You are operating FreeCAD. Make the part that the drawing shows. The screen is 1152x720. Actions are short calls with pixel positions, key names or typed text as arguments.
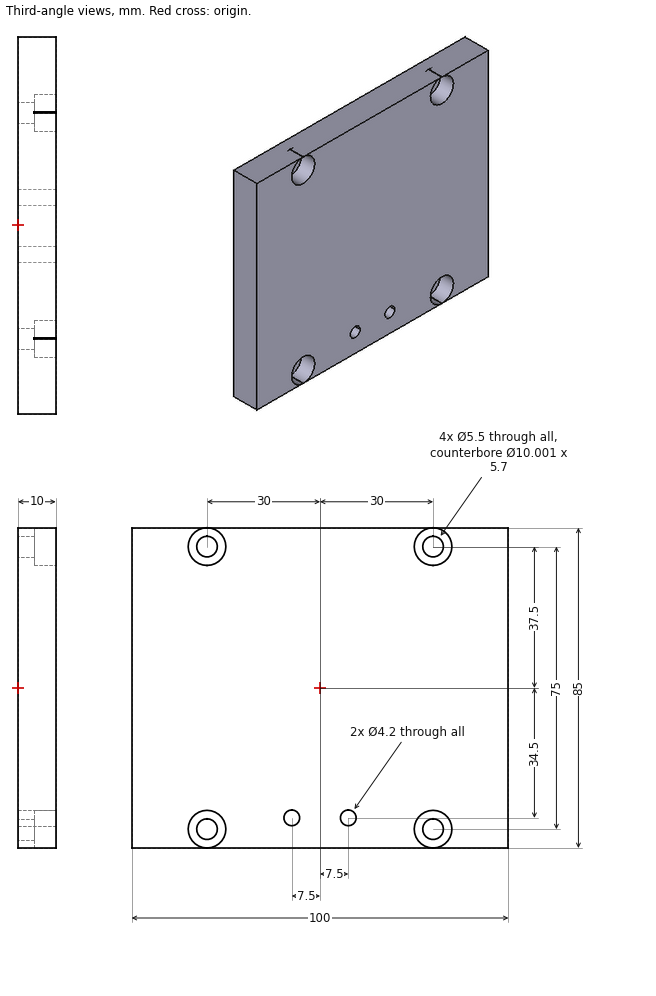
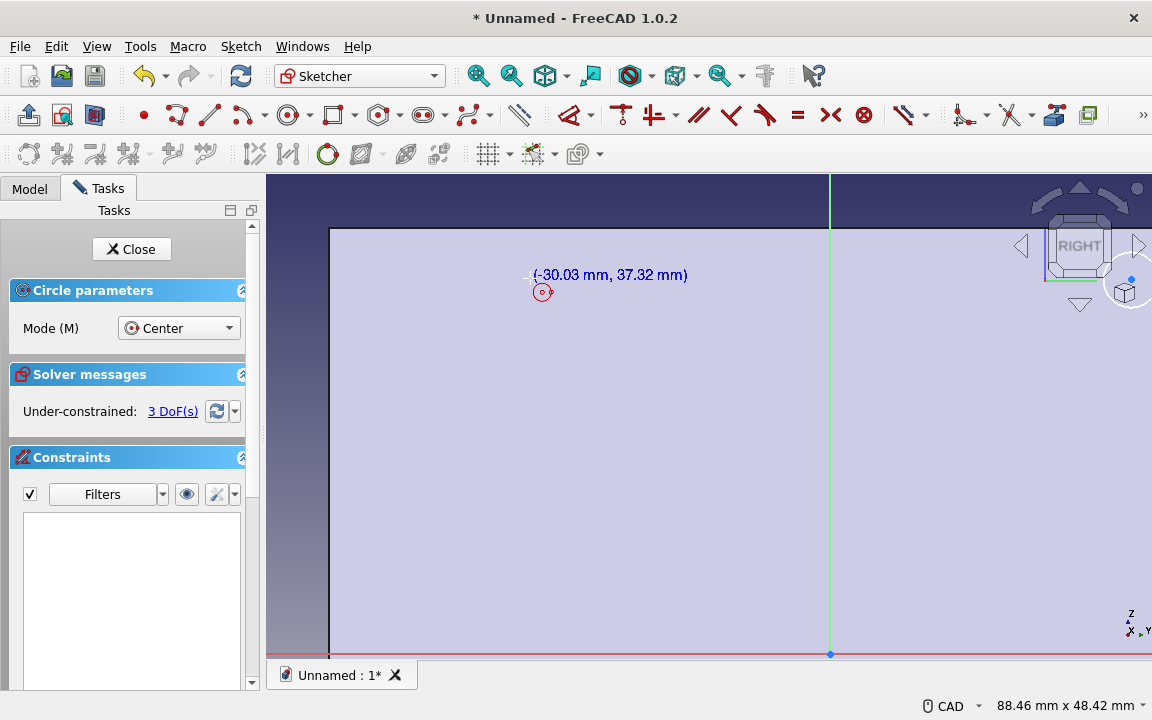
click(530, 279)
click(549, 259)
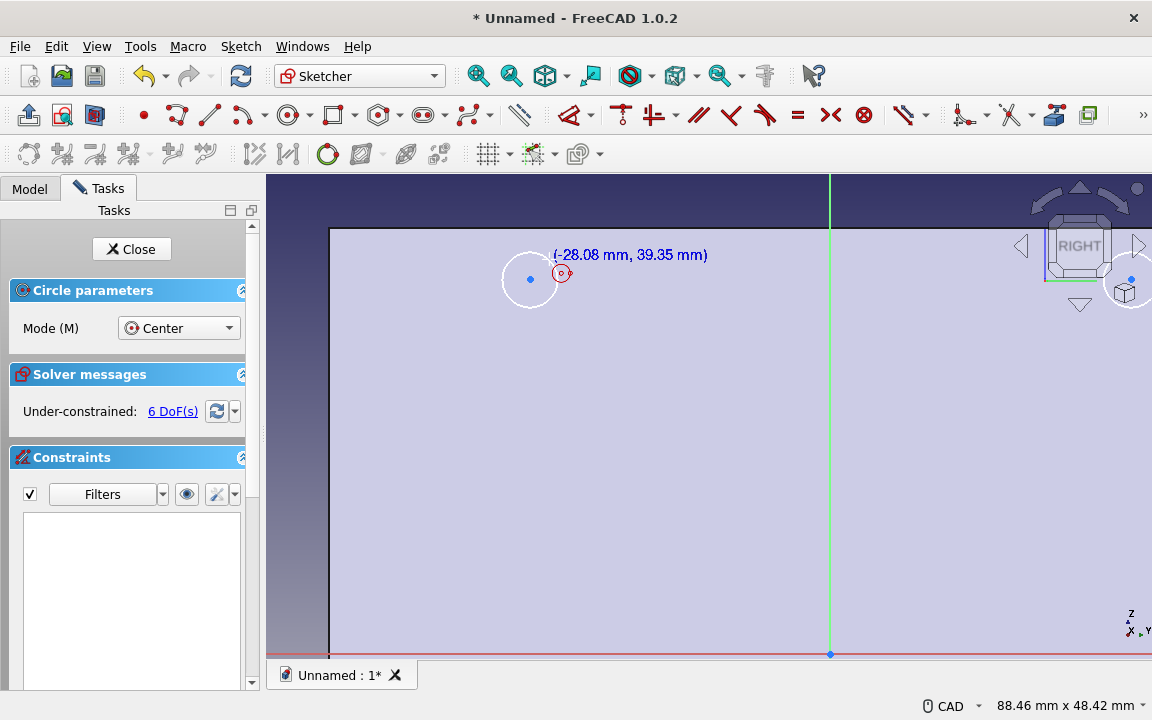
scroll(530, 278, down, 5)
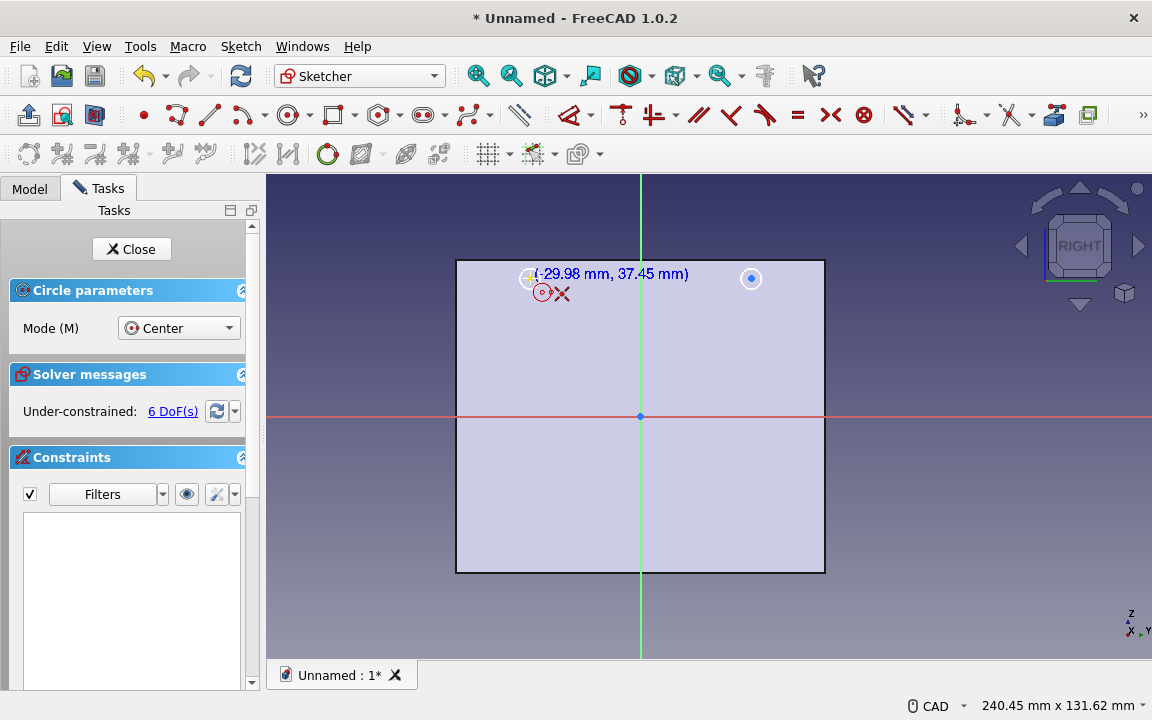
scroll(751, 555, up, 5)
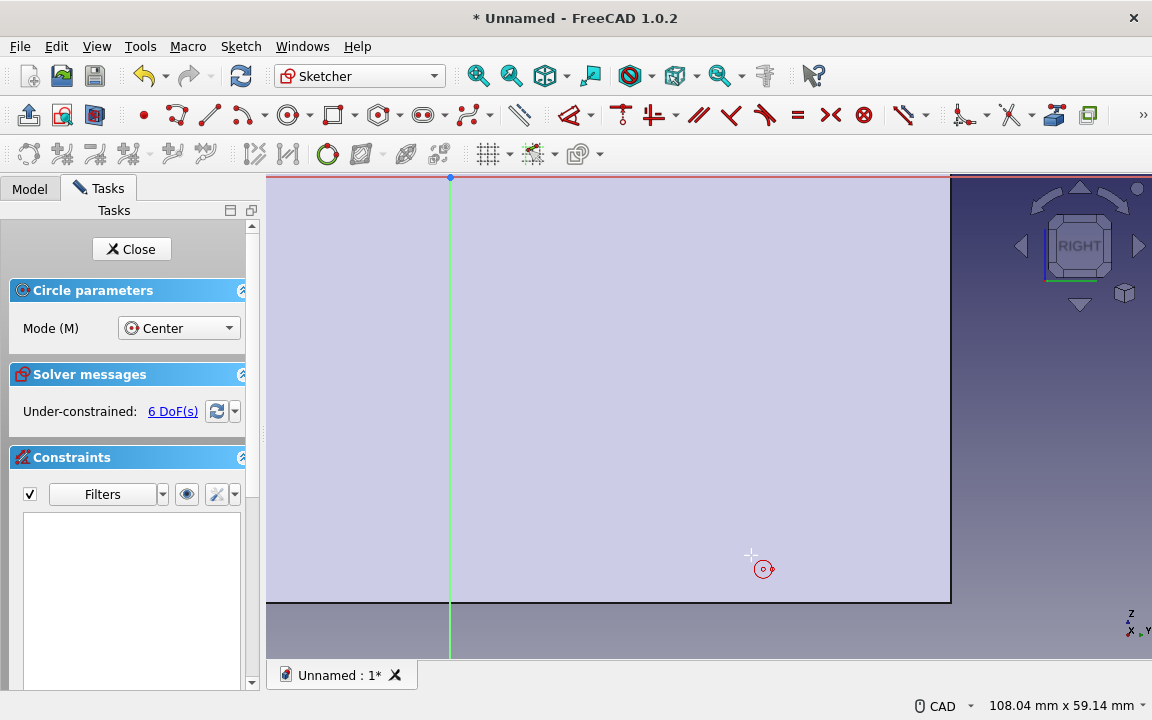
click(751, 553)
click(770, 533)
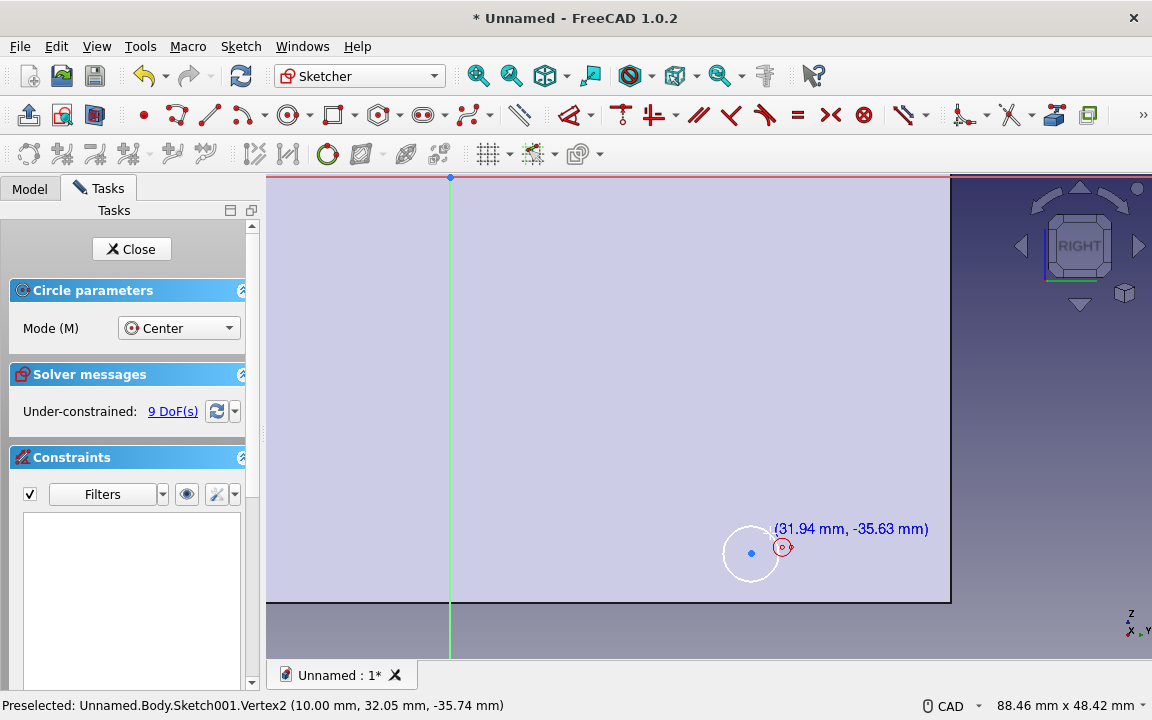
scroll(751, 556, down, 5)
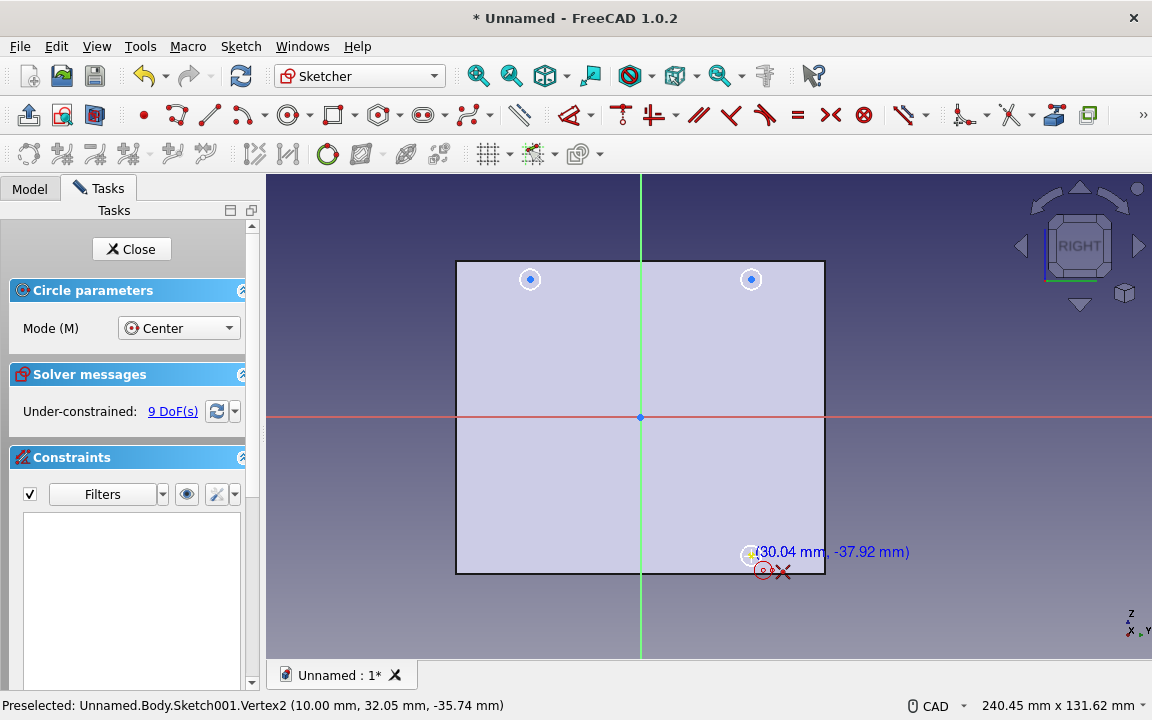
scroll(530, 555, up, 5)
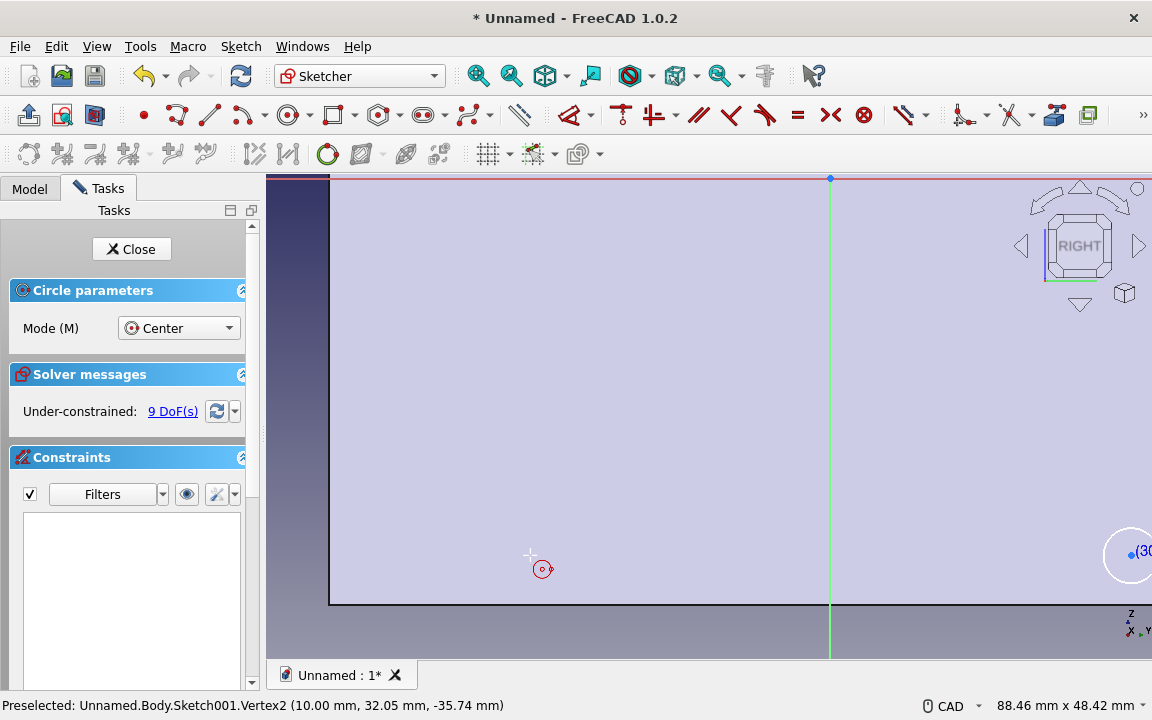
click(530, 554)
click(549, 535)
key(Escape)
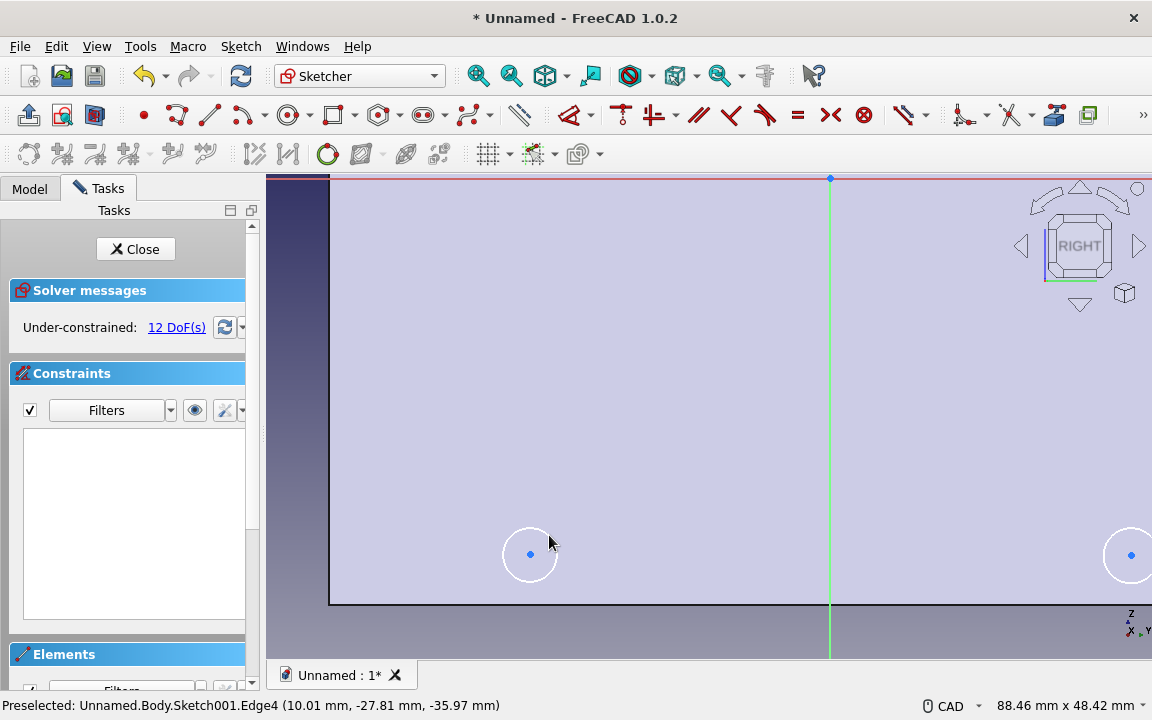
scroll(530, 555, down, 5)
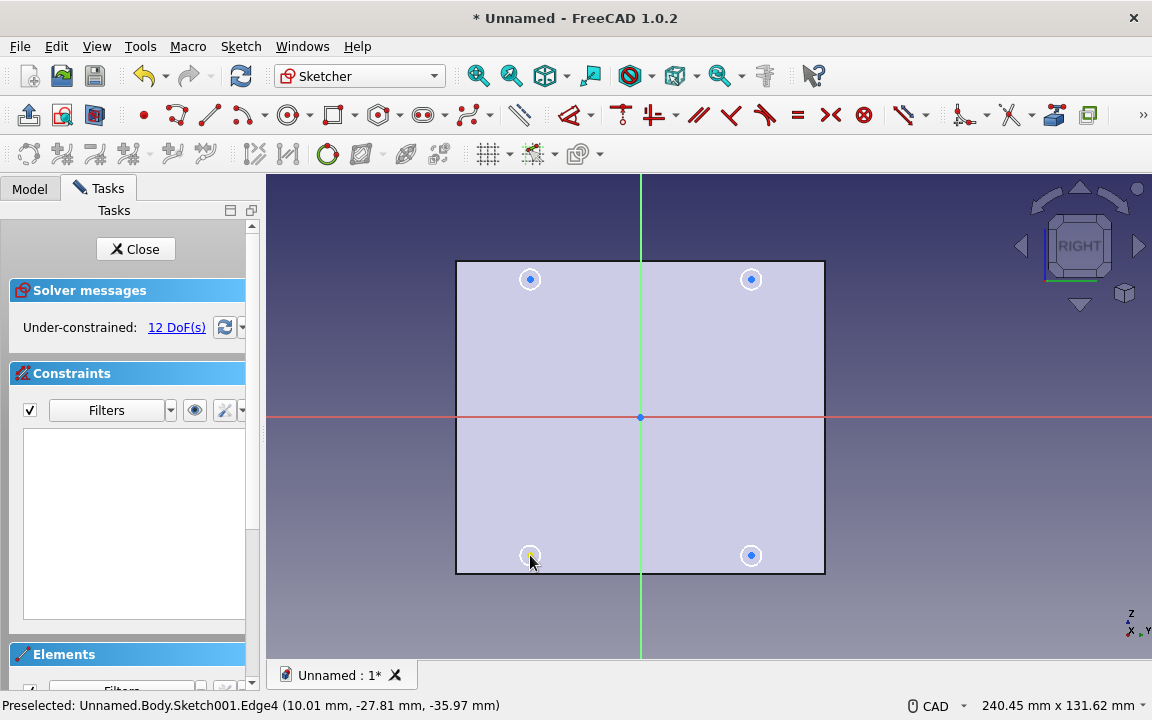
scroll(758, 272, up, 2)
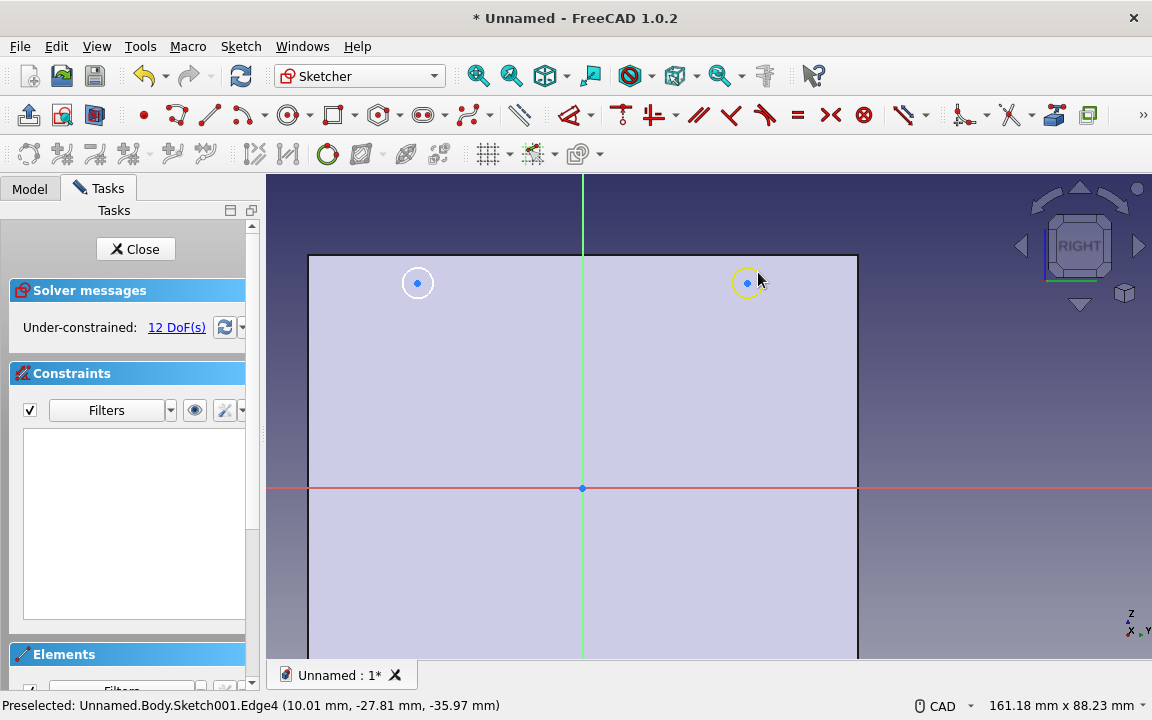
click(758, 272)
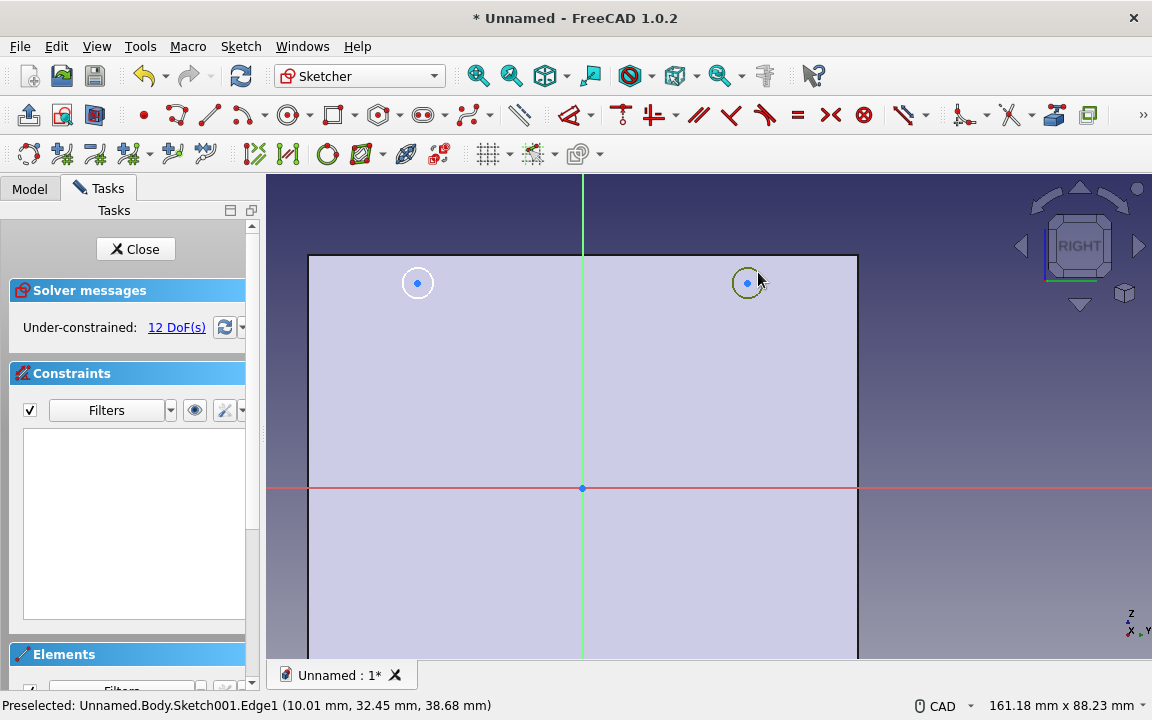
click(429, 272)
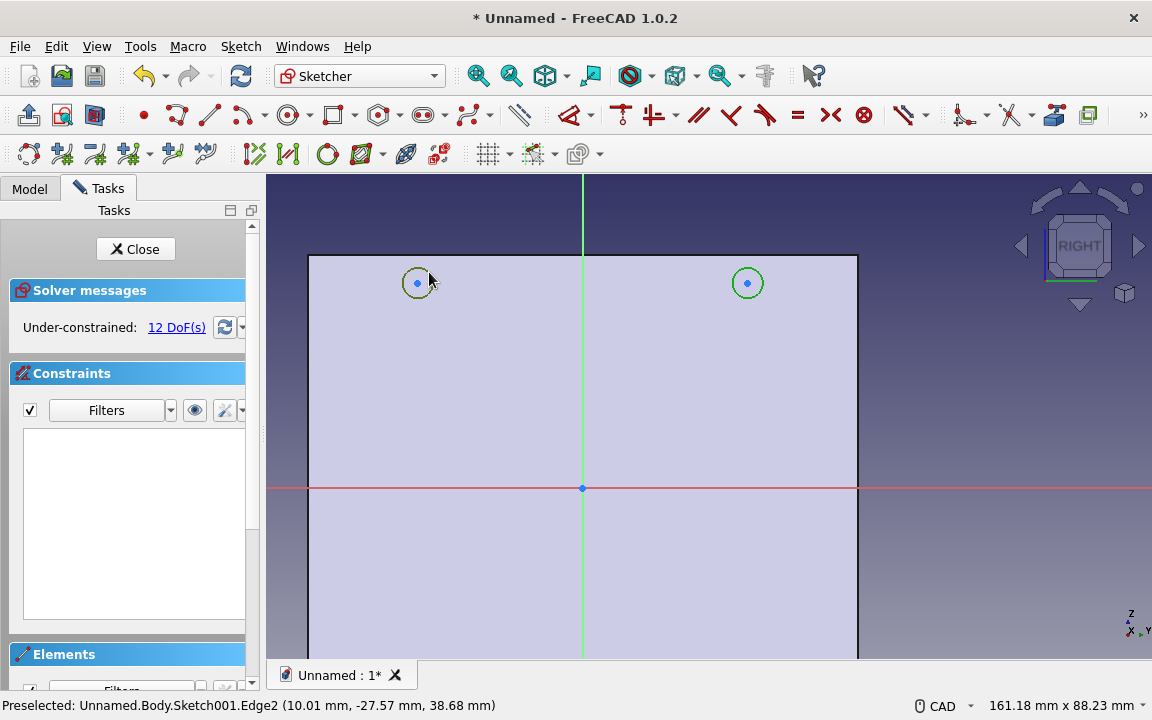
scroll(758, 270, down, 2)